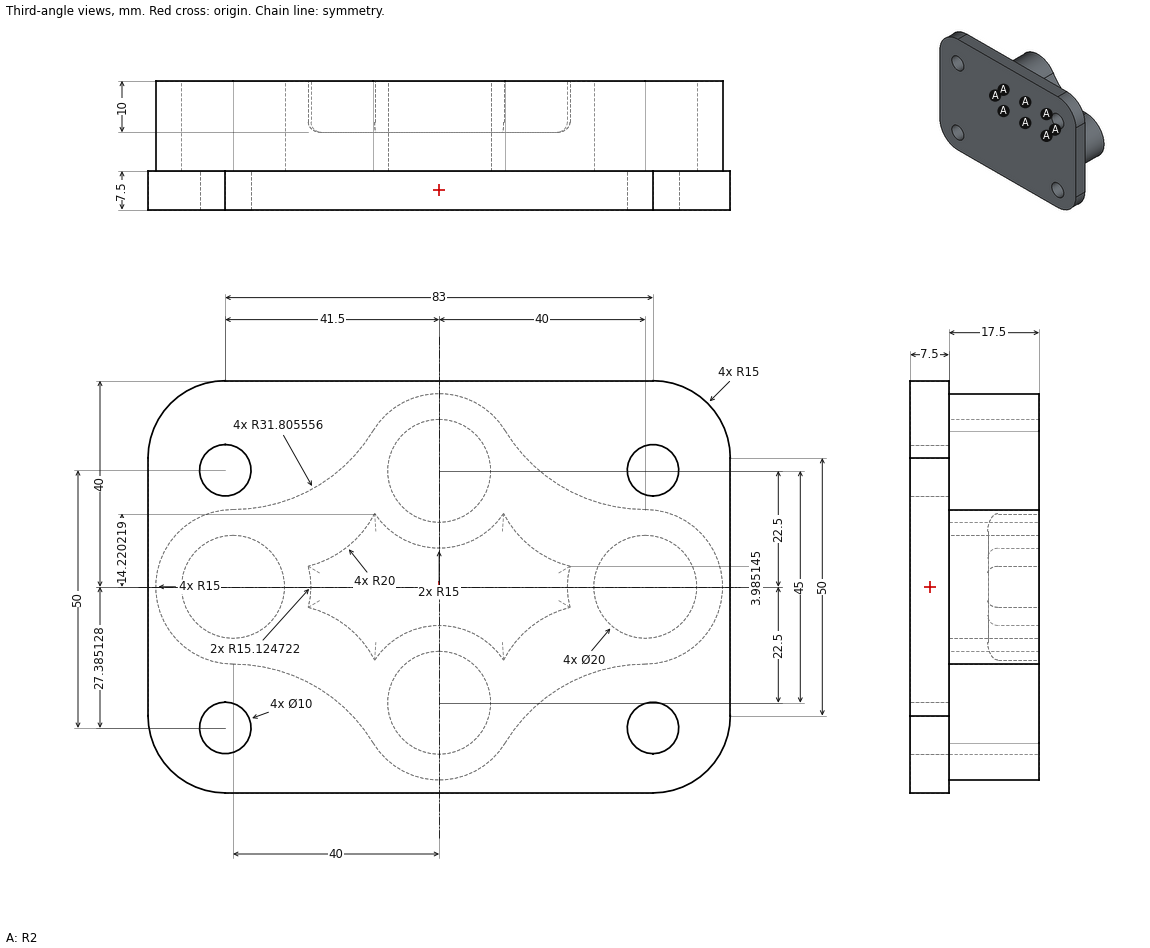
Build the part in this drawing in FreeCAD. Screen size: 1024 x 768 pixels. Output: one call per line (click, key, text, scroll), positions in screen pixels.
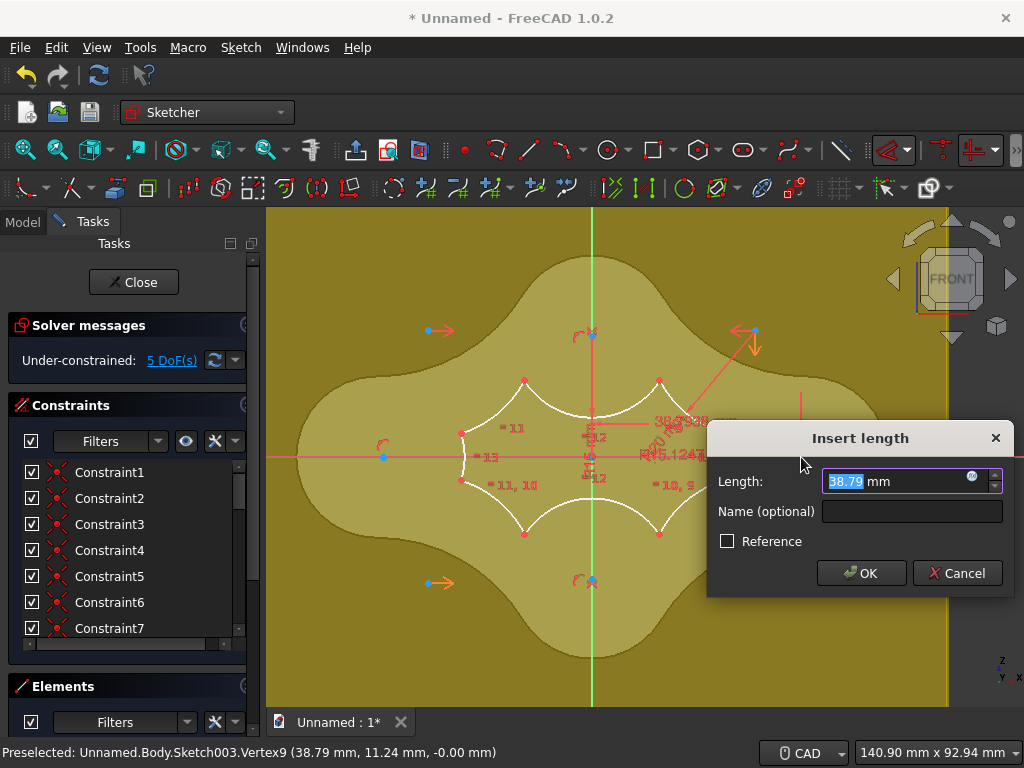
text(40)
key(Return)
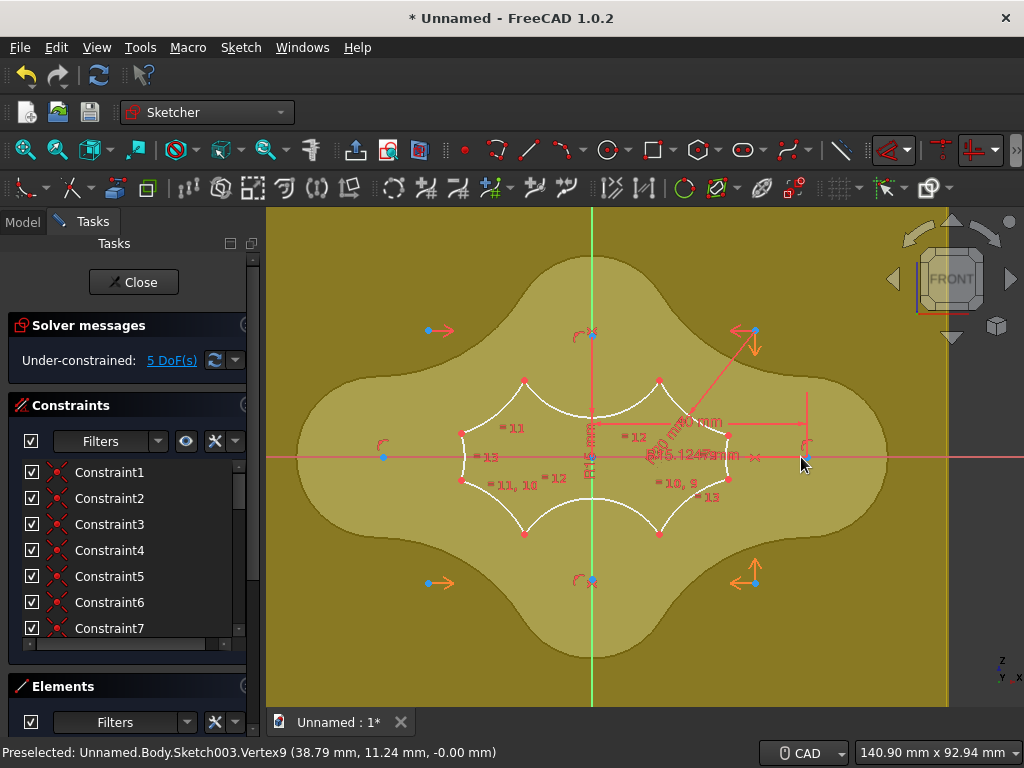
click(383, 457)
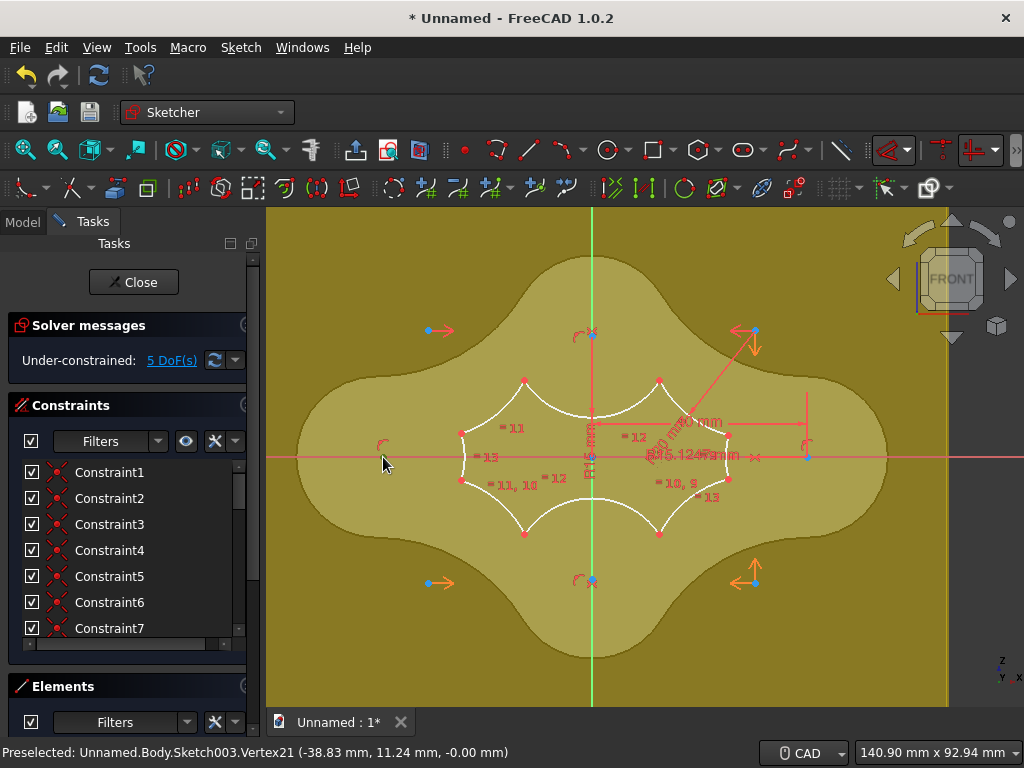
click(910, 150)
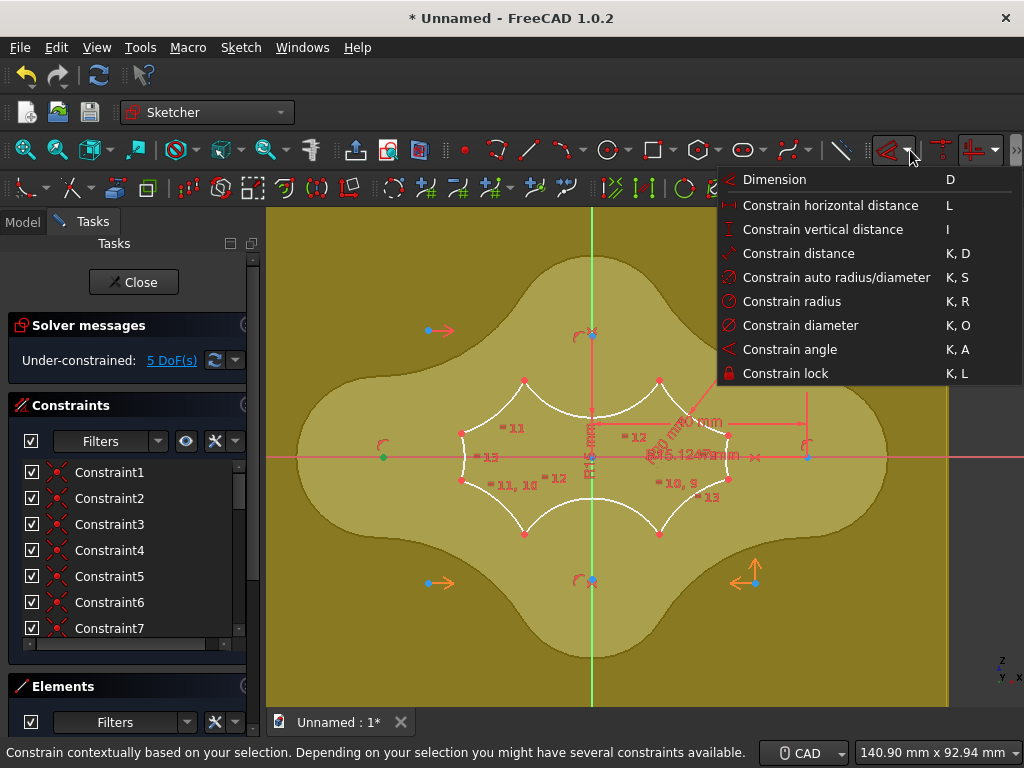
click(870, 205)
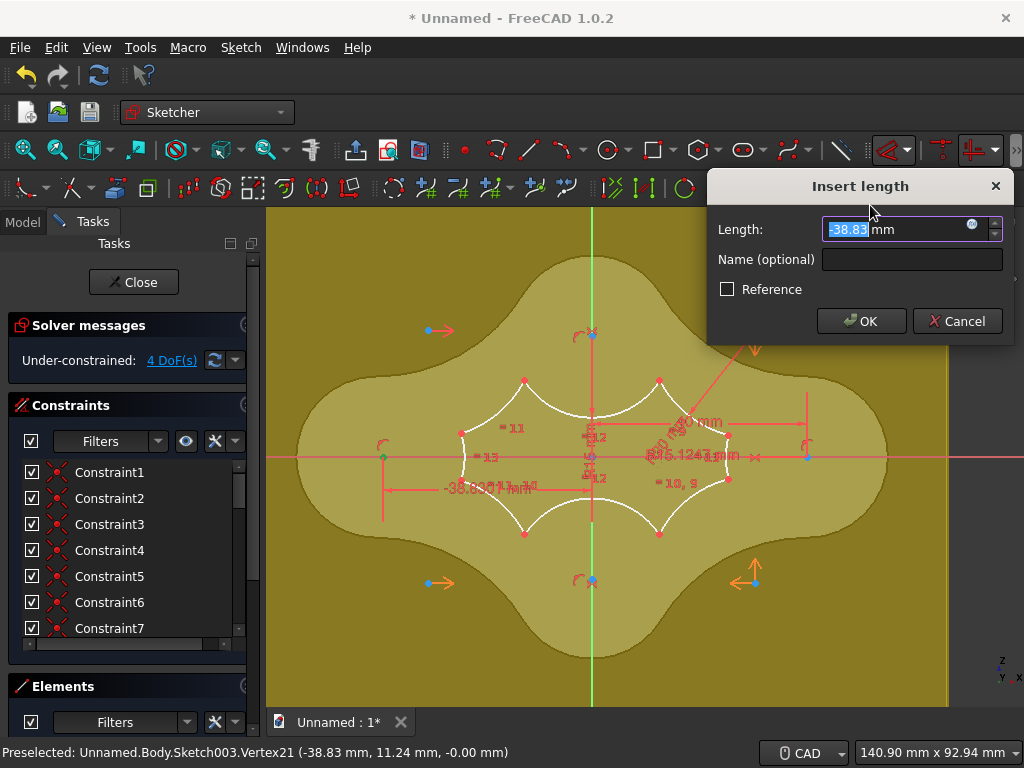
text(-40)
key(Return)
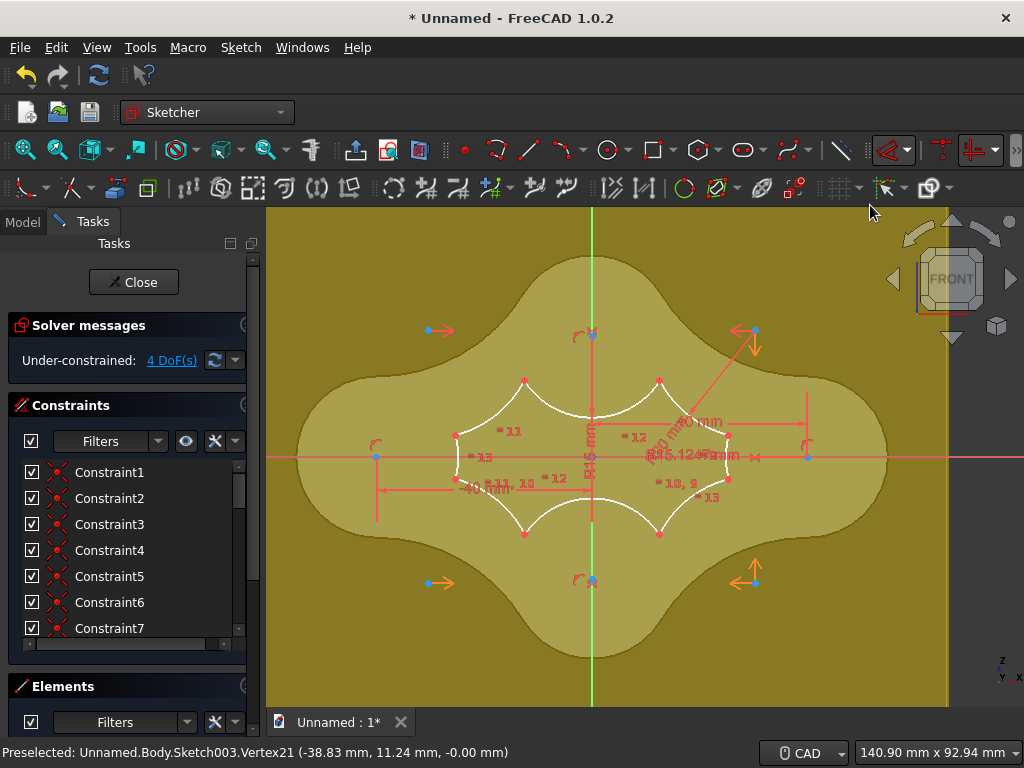
click(592, 337)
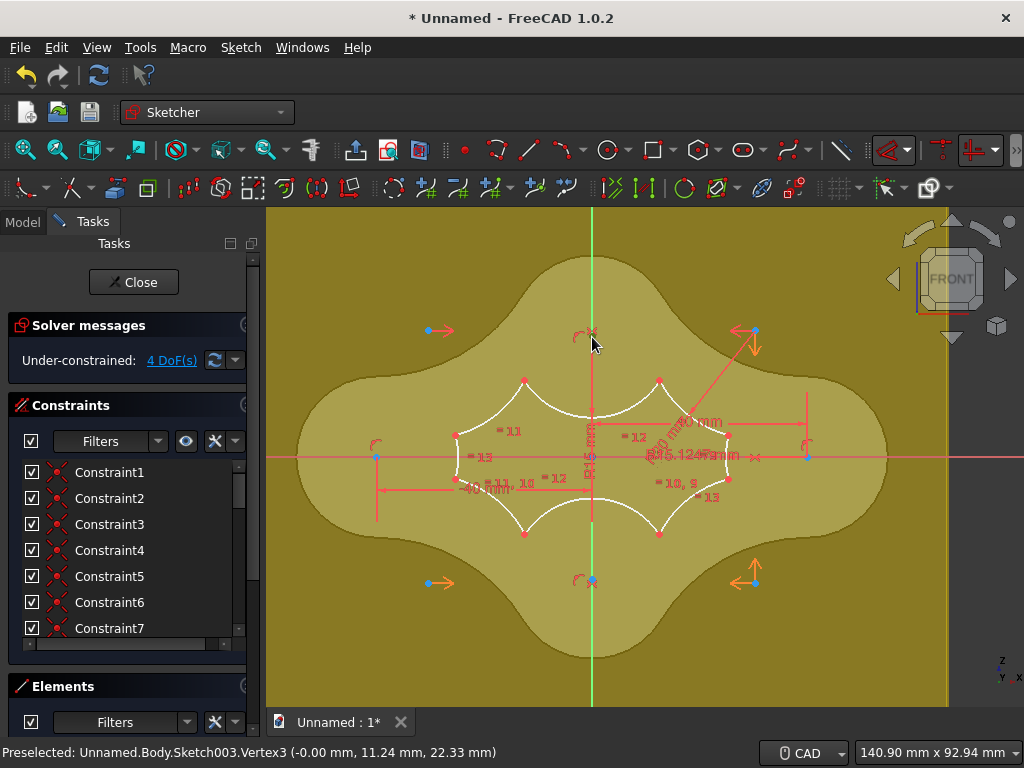
click(910, 150)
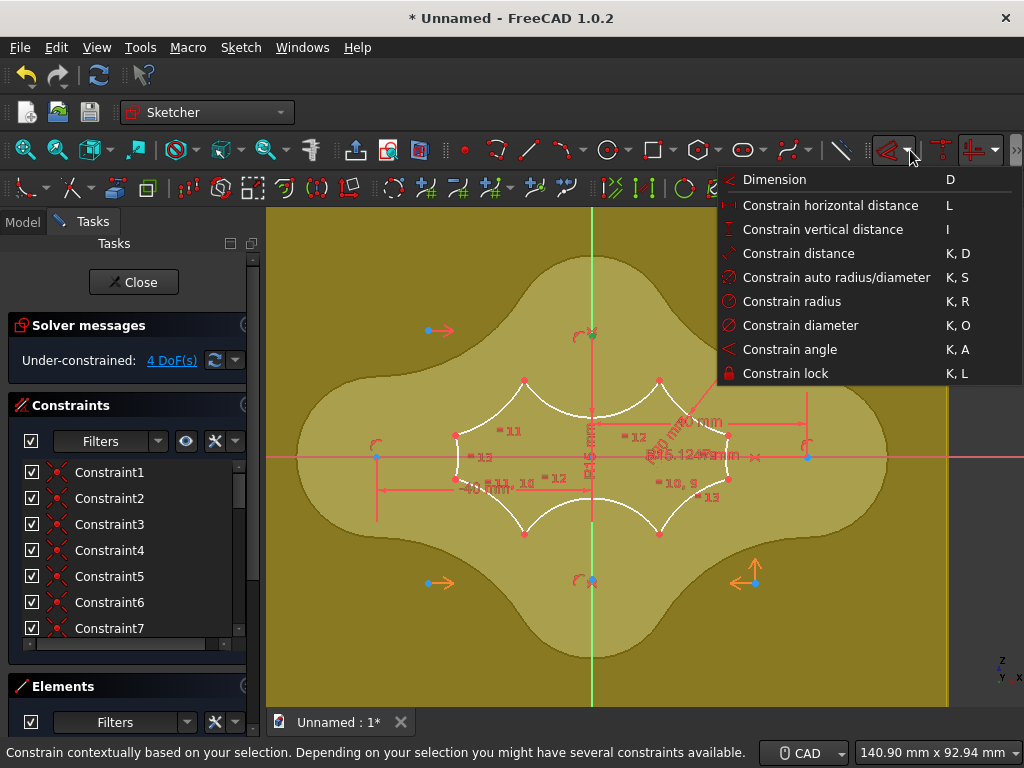
click(870, 229)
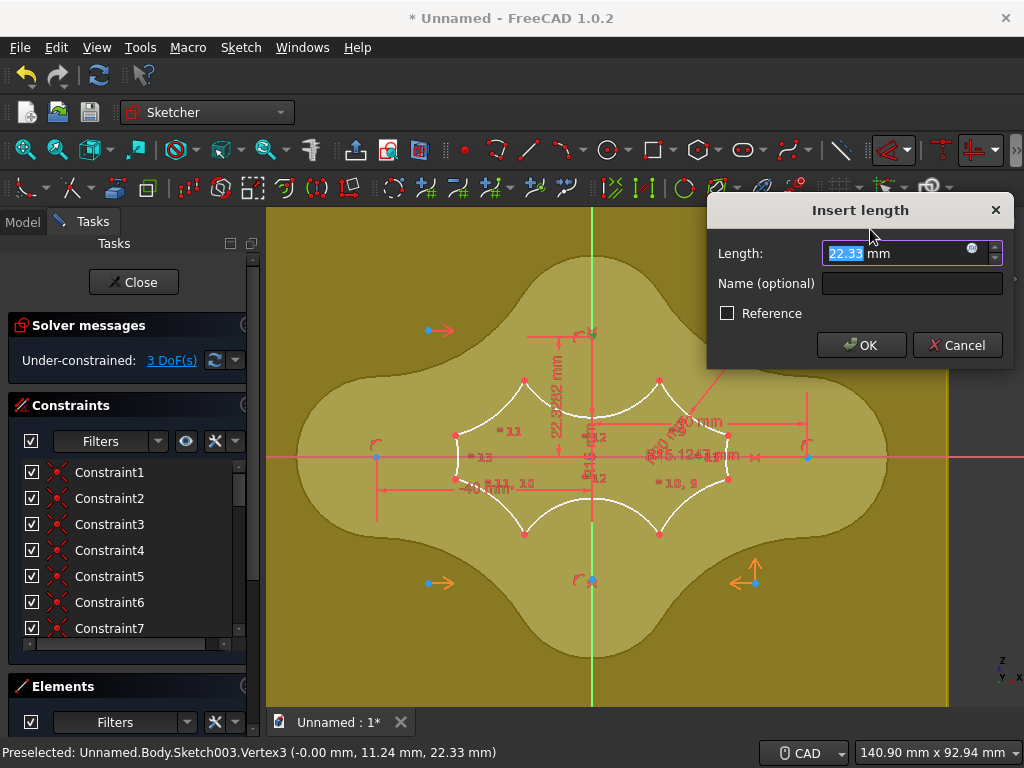
text(22.5)
key(Return)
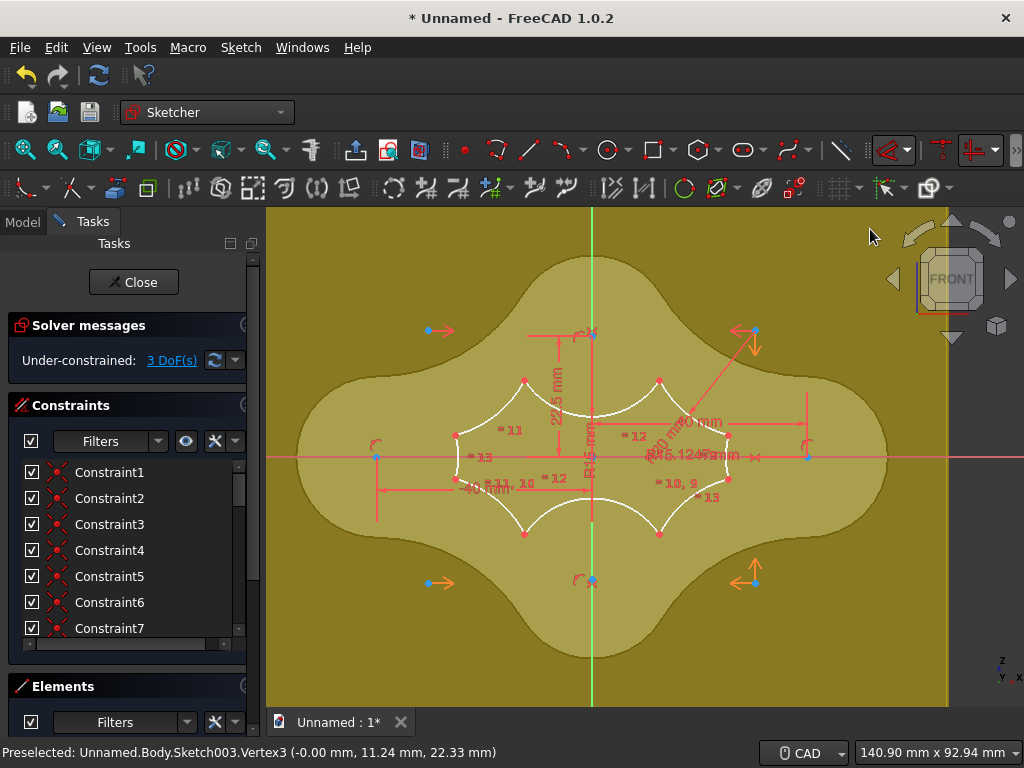
click(592, 579)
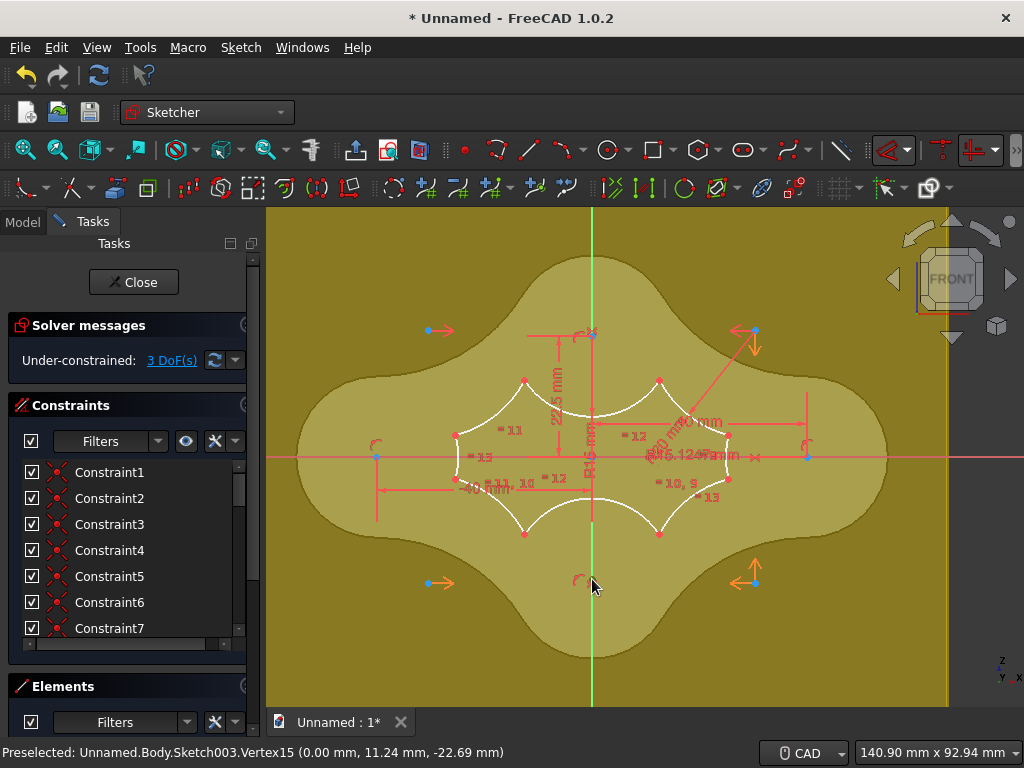
click(910, 150)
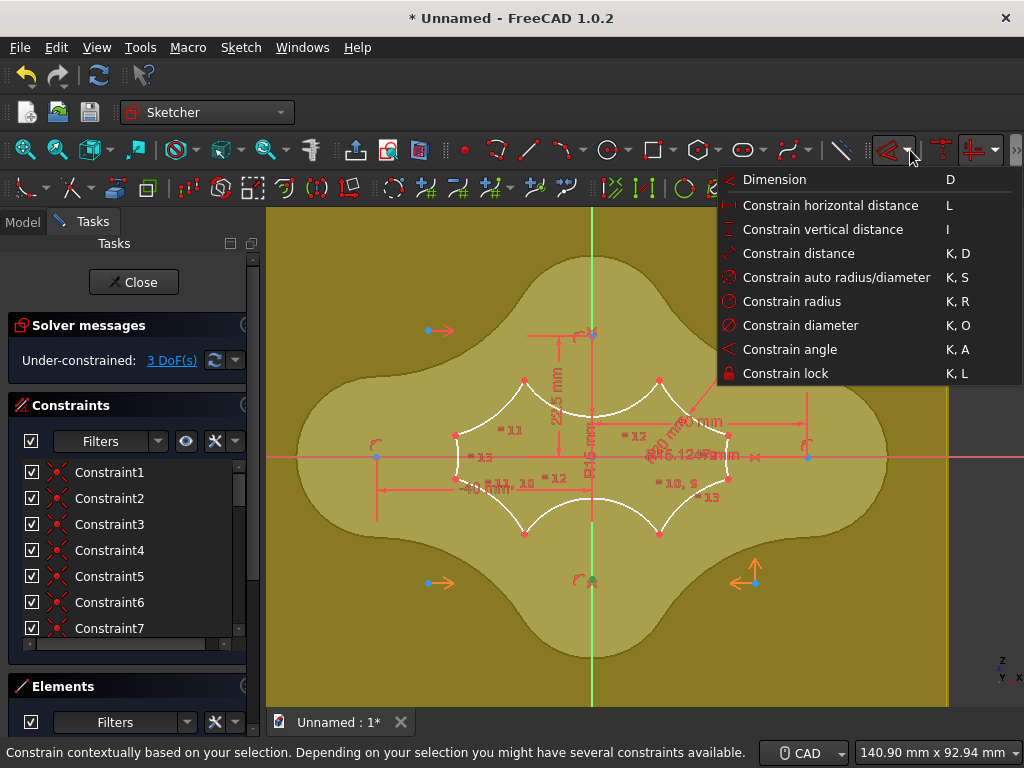
click(870, 229)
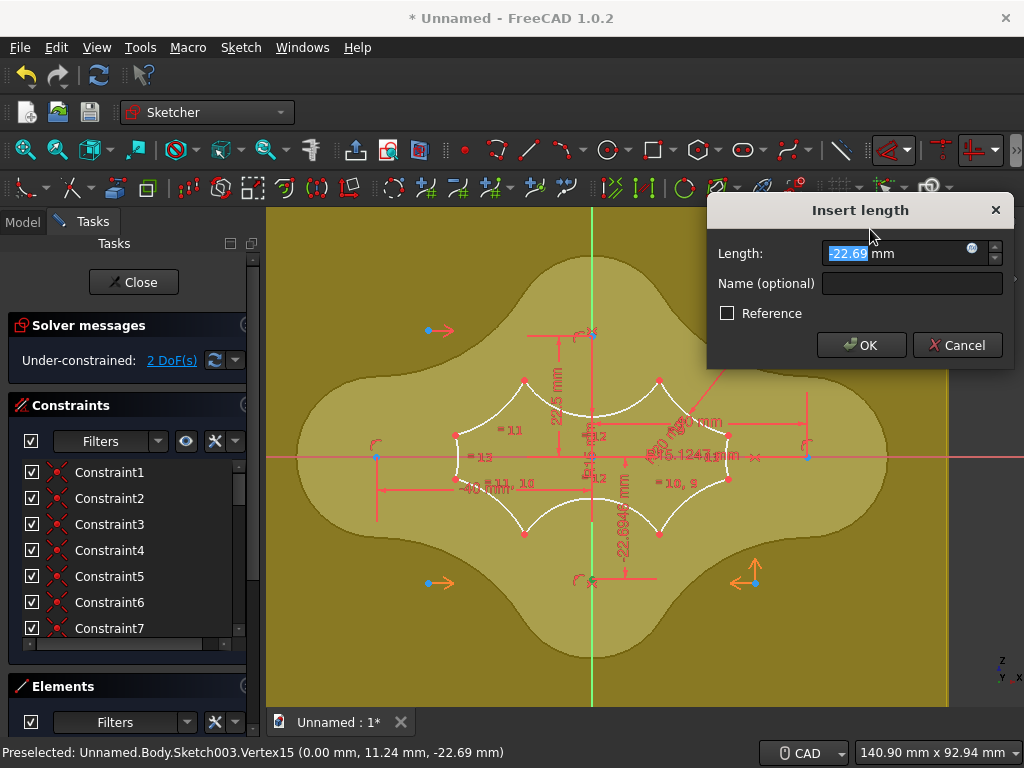
text(-22.5)
key(Return)